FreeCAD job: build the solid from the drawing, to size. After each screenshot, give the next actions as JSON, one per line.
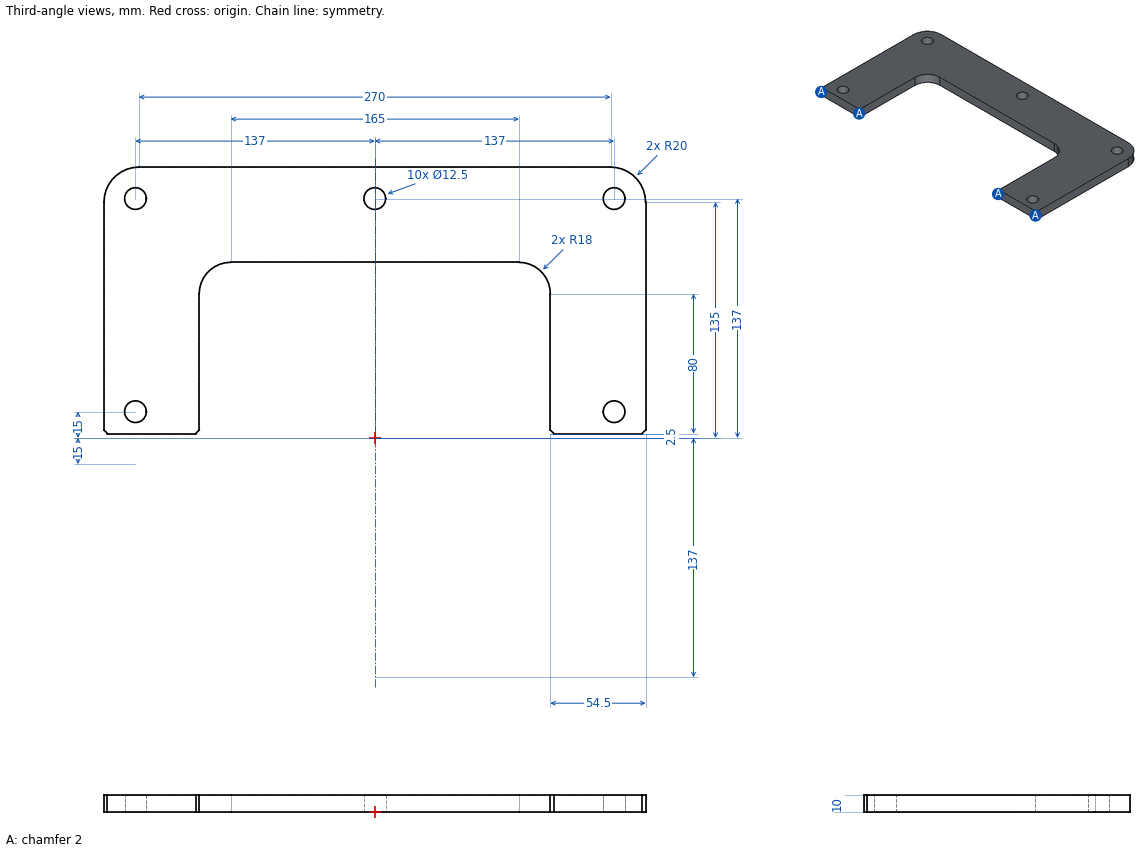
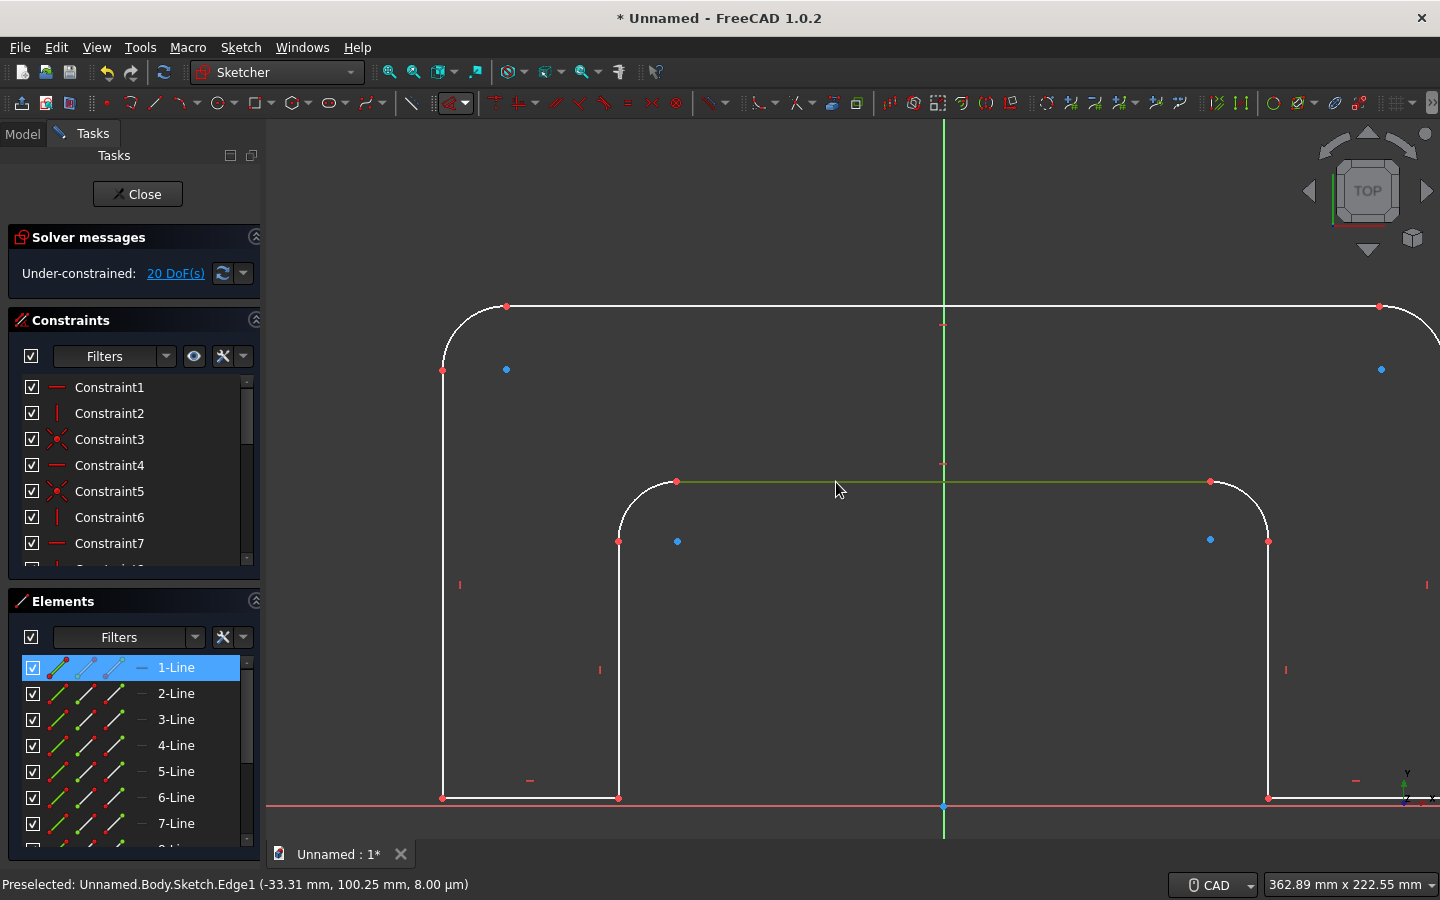
{"action": "left_click", "coordinate": [1263, 514]}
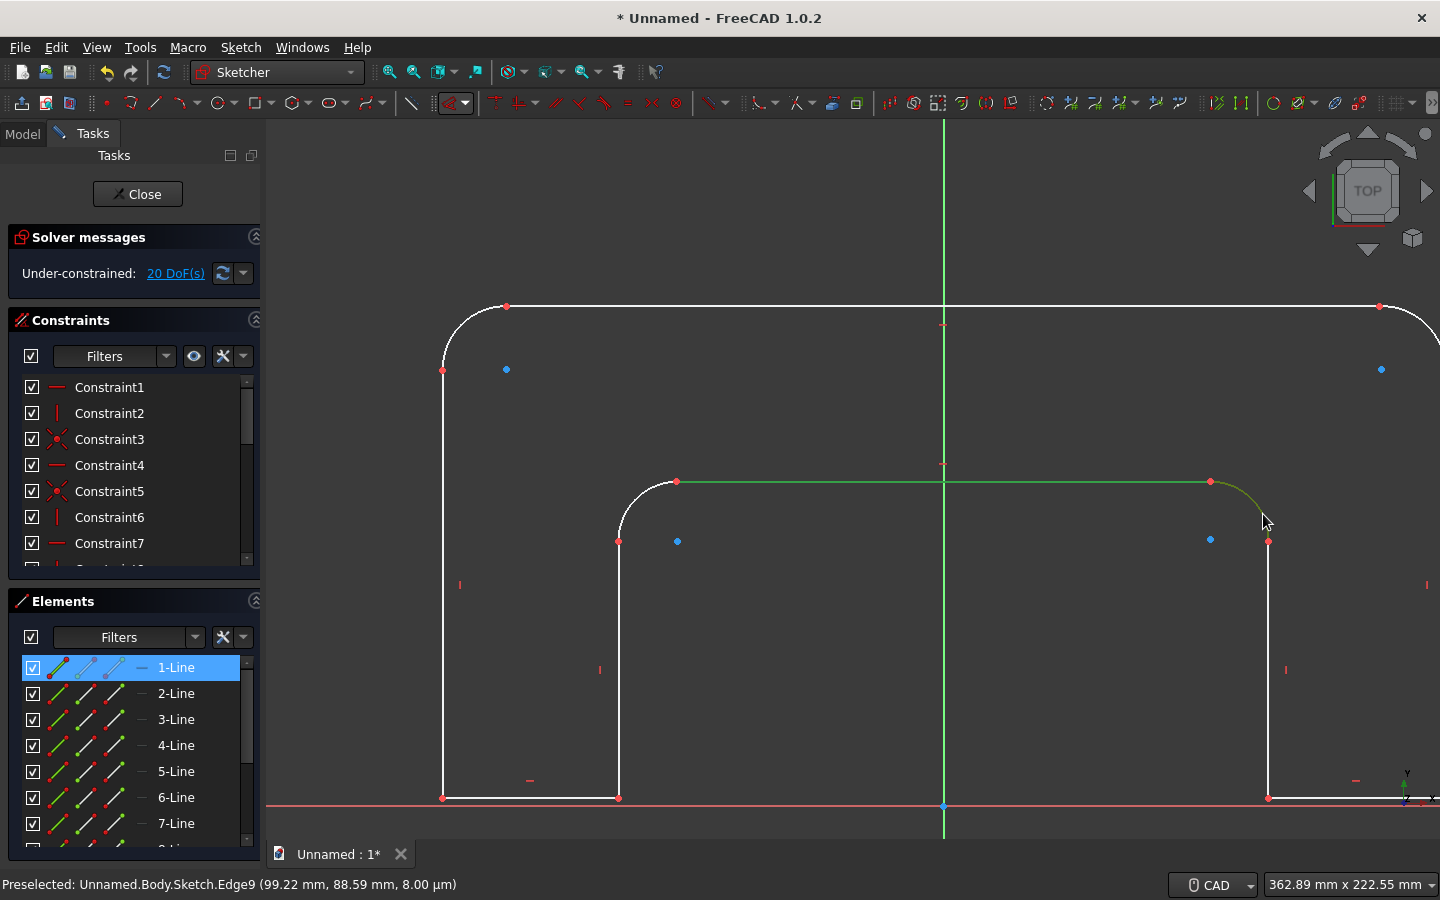
{"action": "key", "text": "t"}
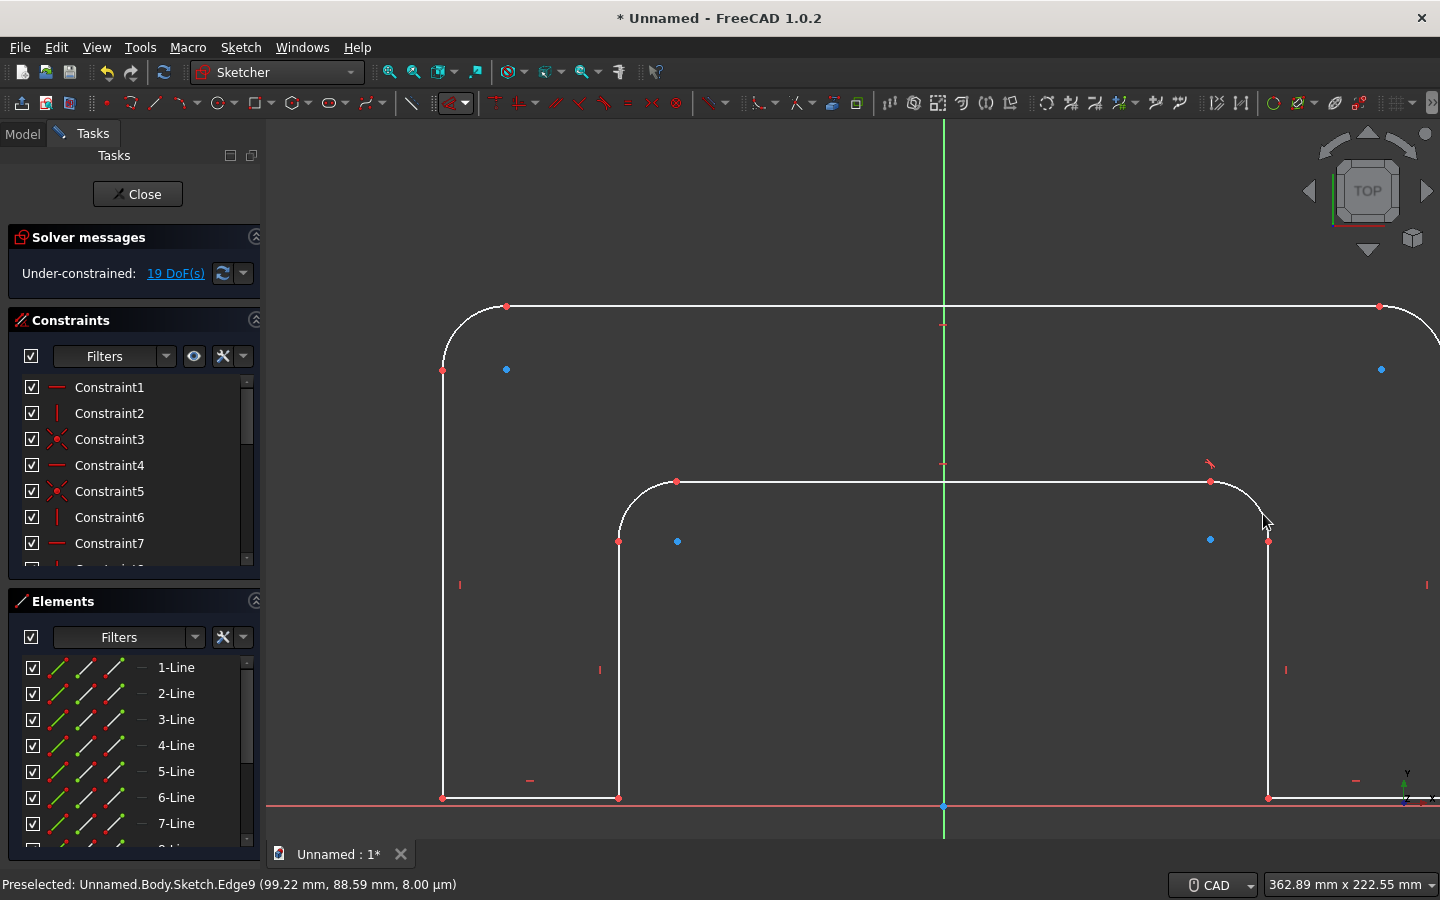
{"action": "left_click", "coordinate": [836, 482]}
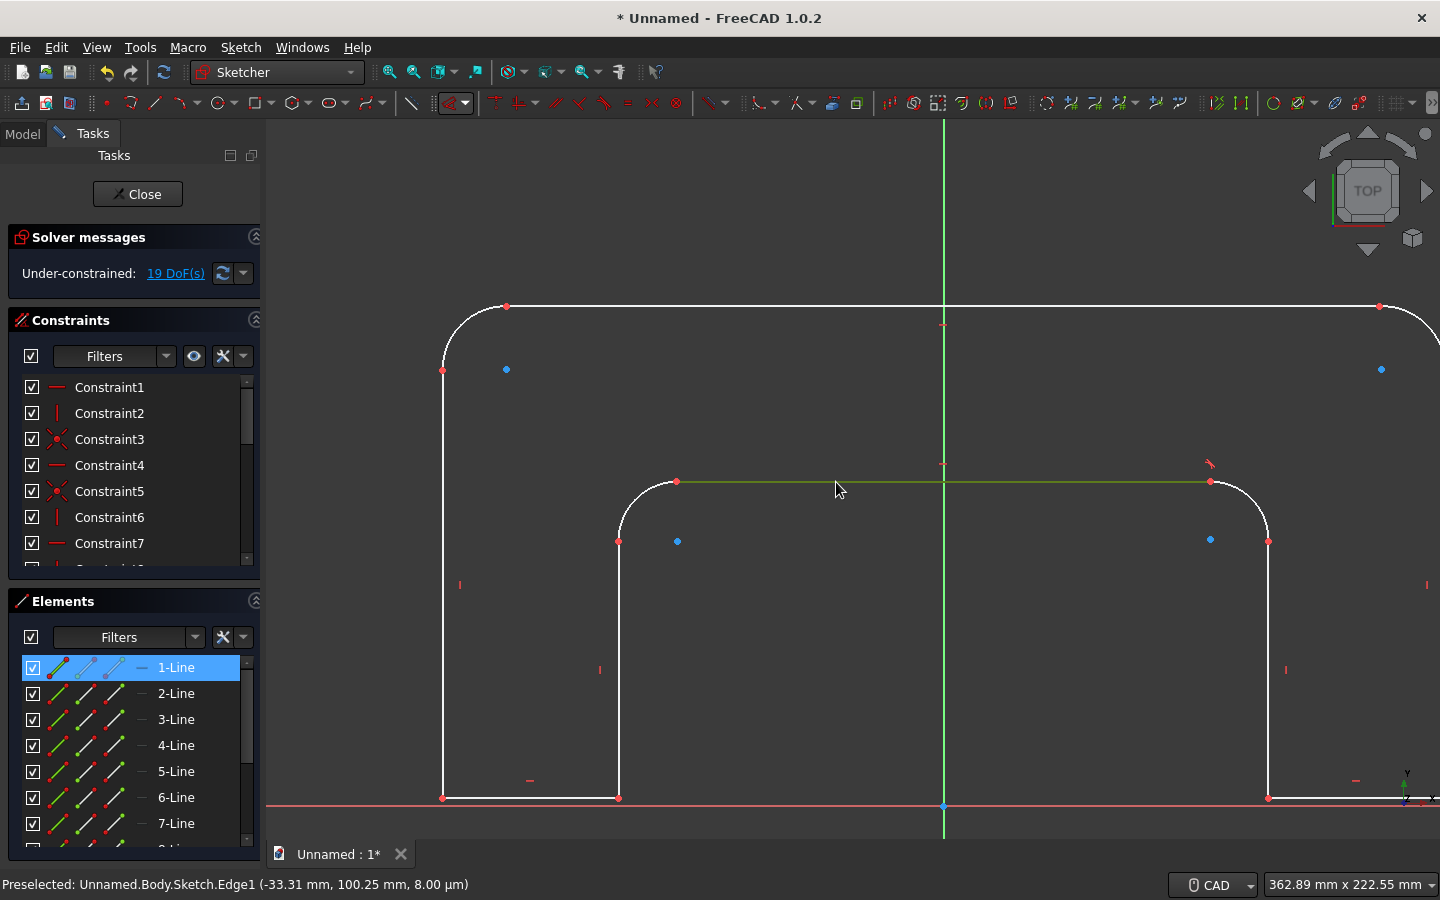
{"action": "left_click", "coordinate": [650, 489]}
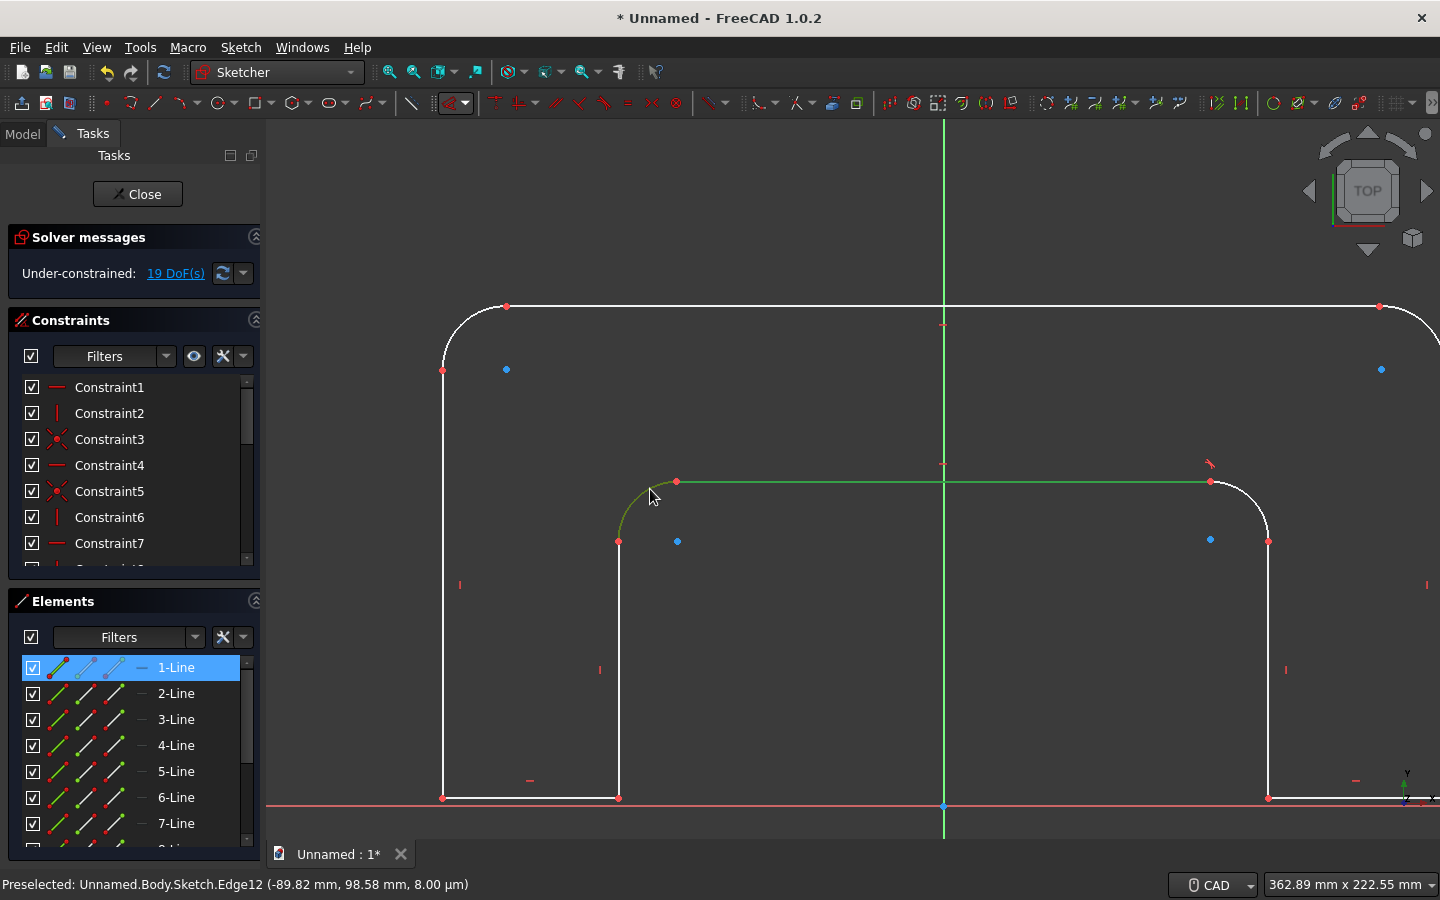
{"action": "key", "text": "t"}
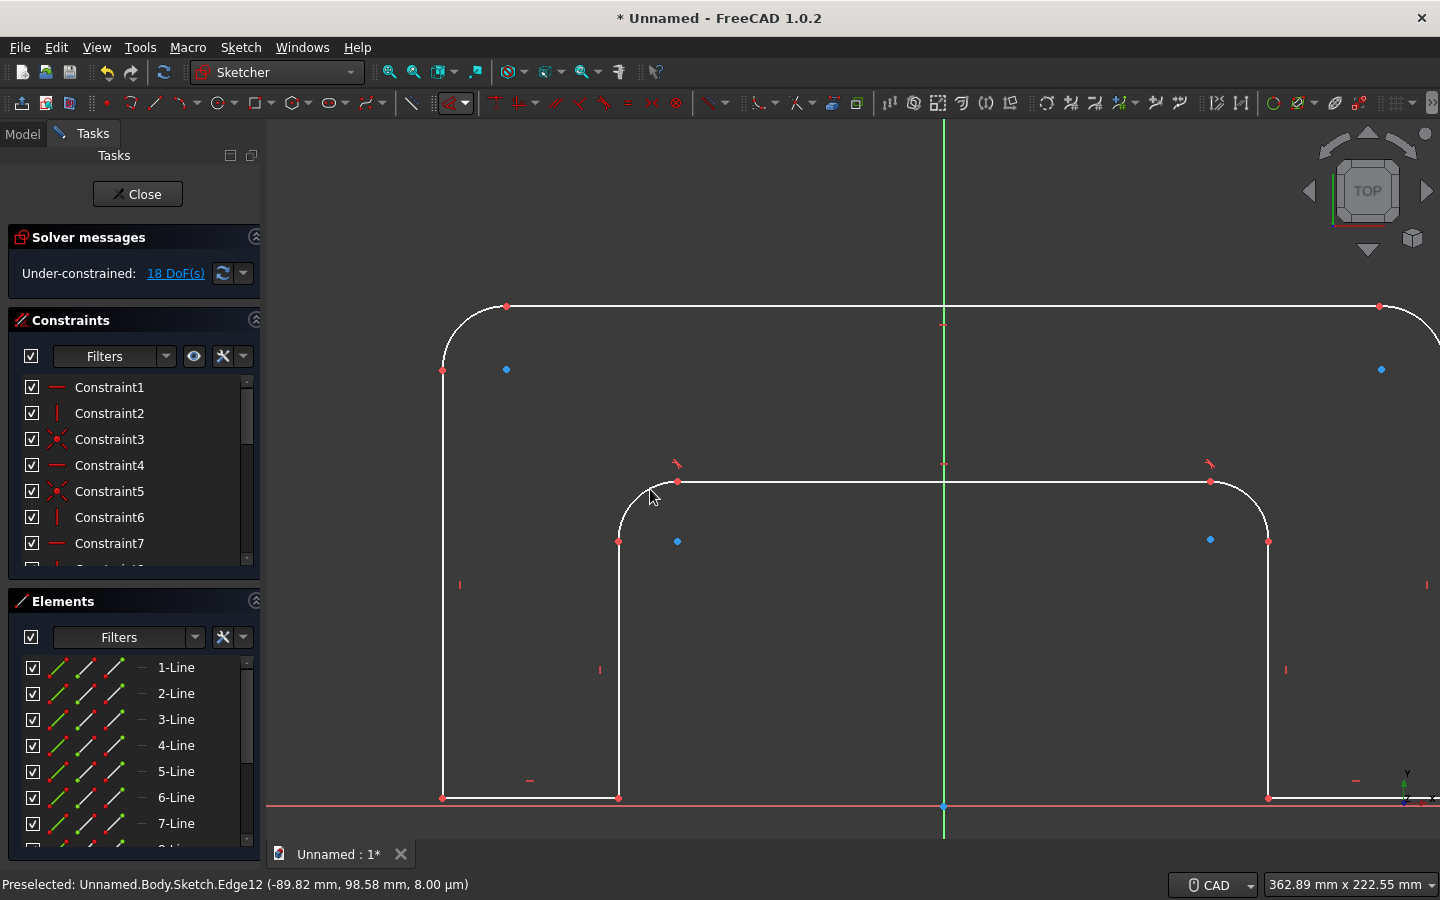
{"action": "left_click", "coordinate": [1268, 618]}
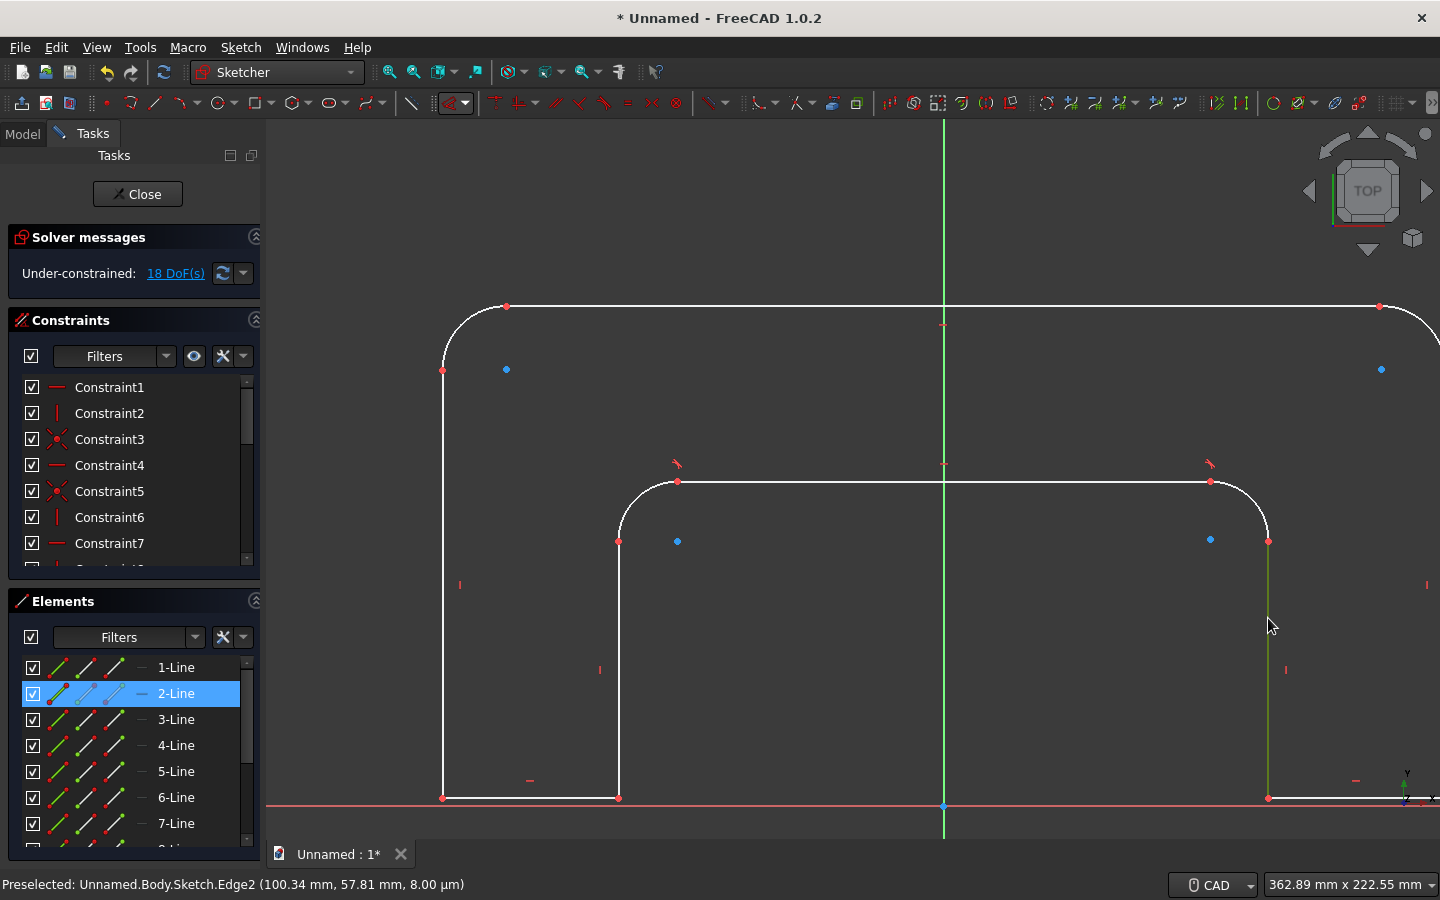
{"action": "left_click", "coordinate": [1263, 514]}